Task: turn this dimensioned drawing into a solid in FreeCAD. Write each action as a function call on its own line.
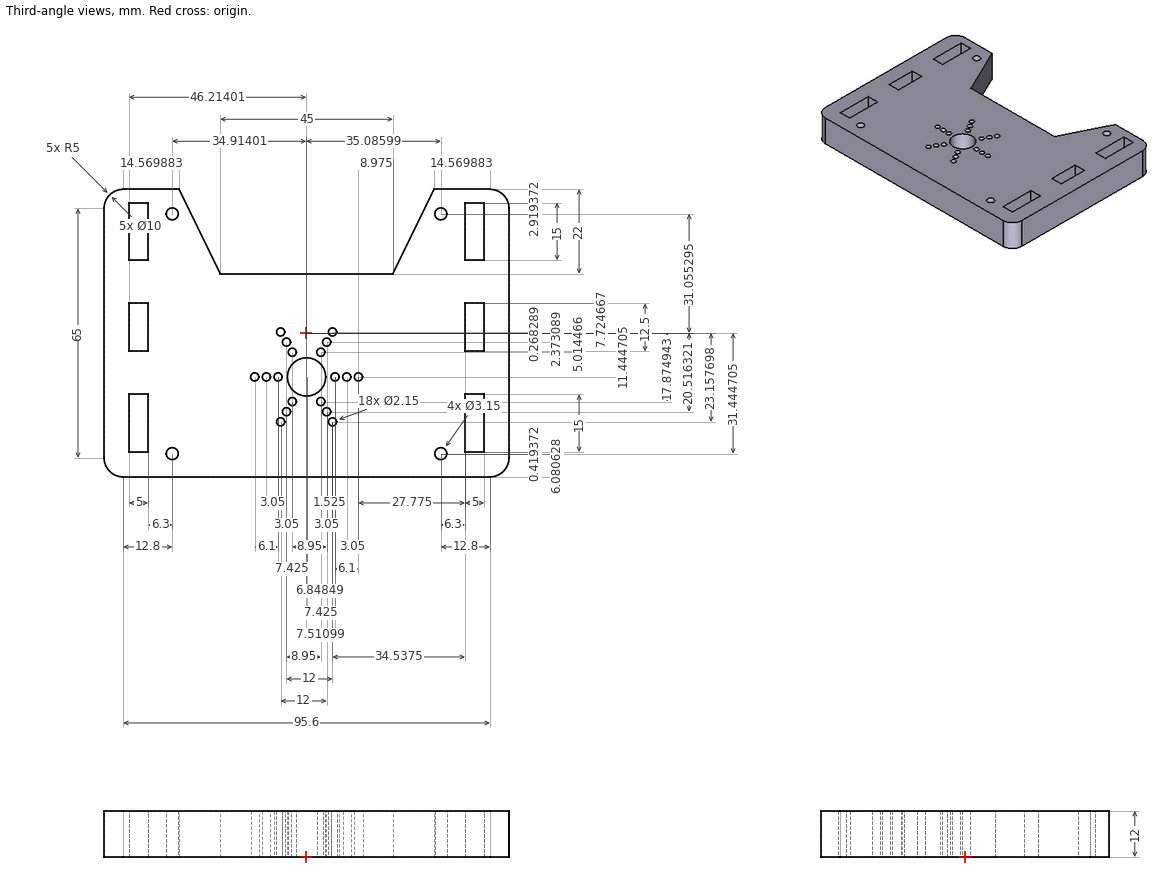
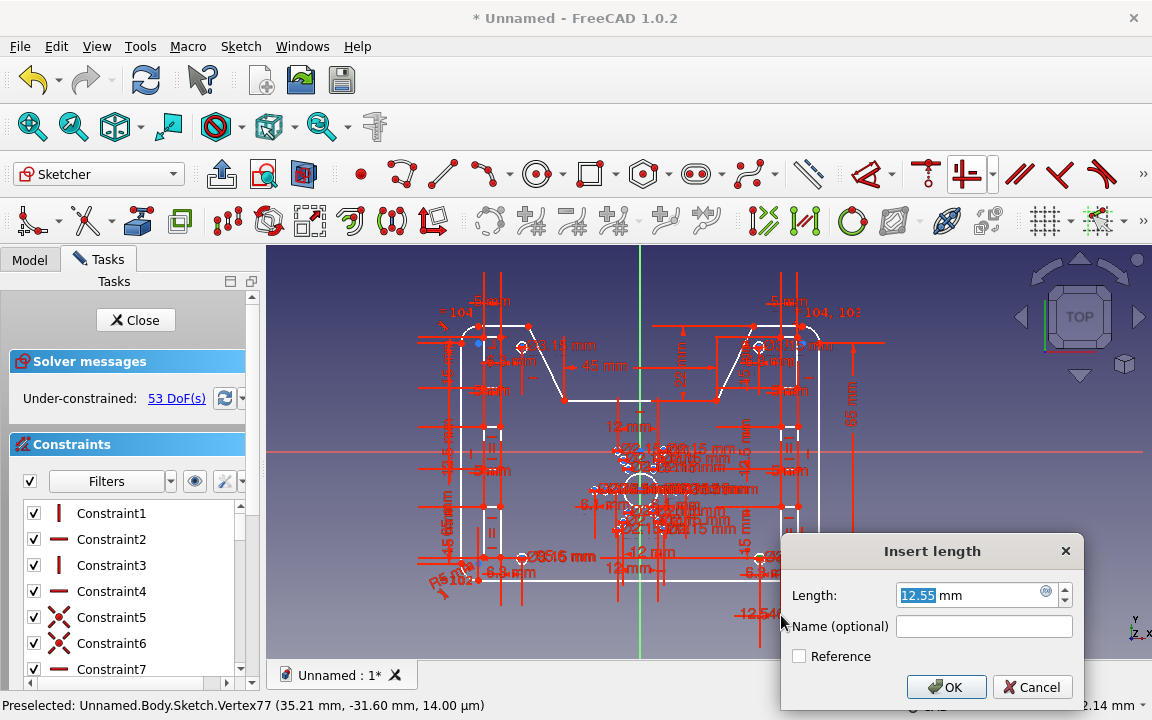
text(12.8)
key(Return)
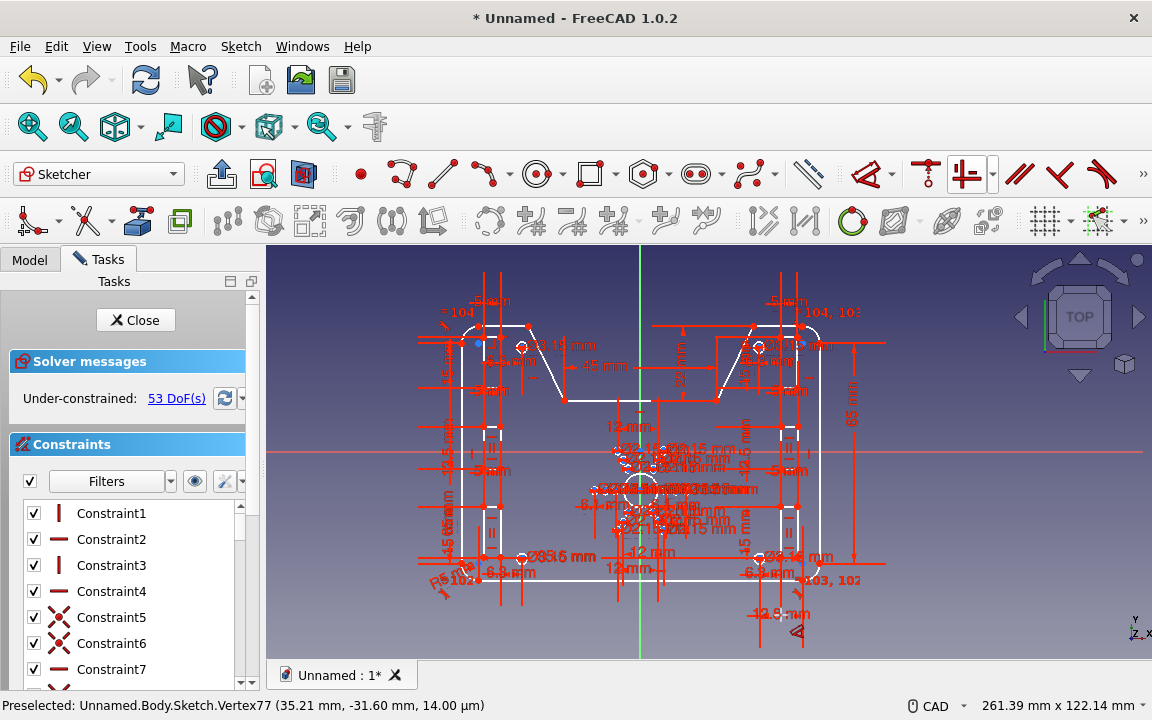
scroll(664, 531, up, 7)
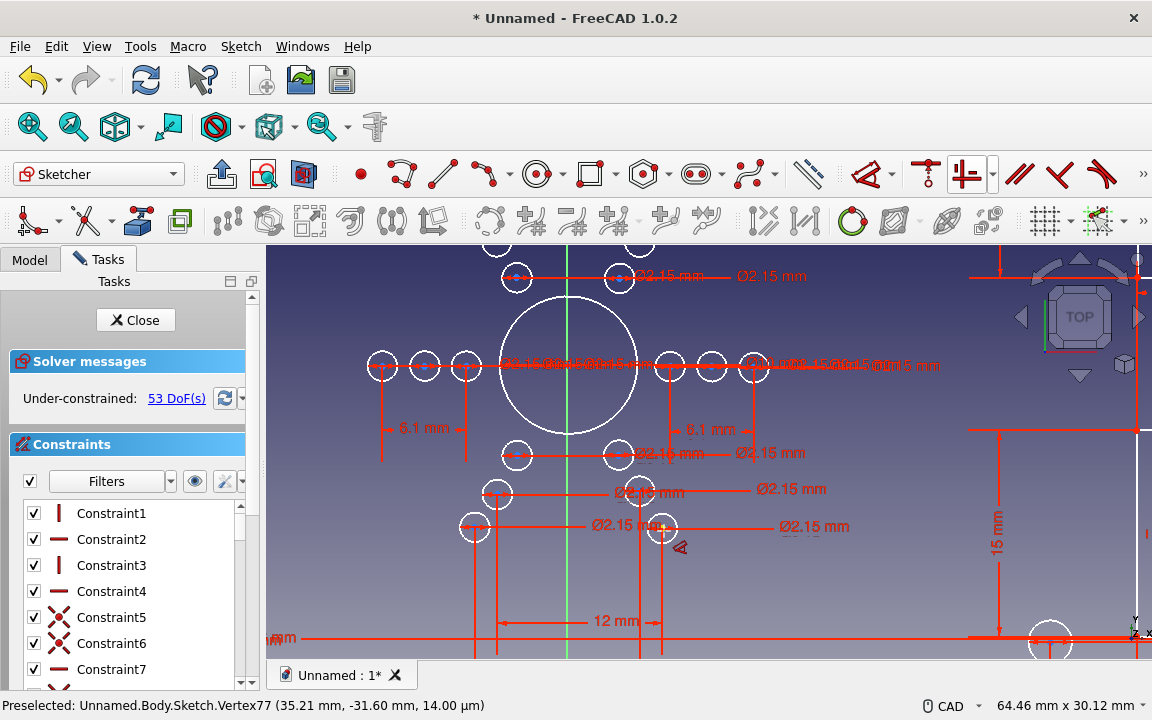
click(662, 529)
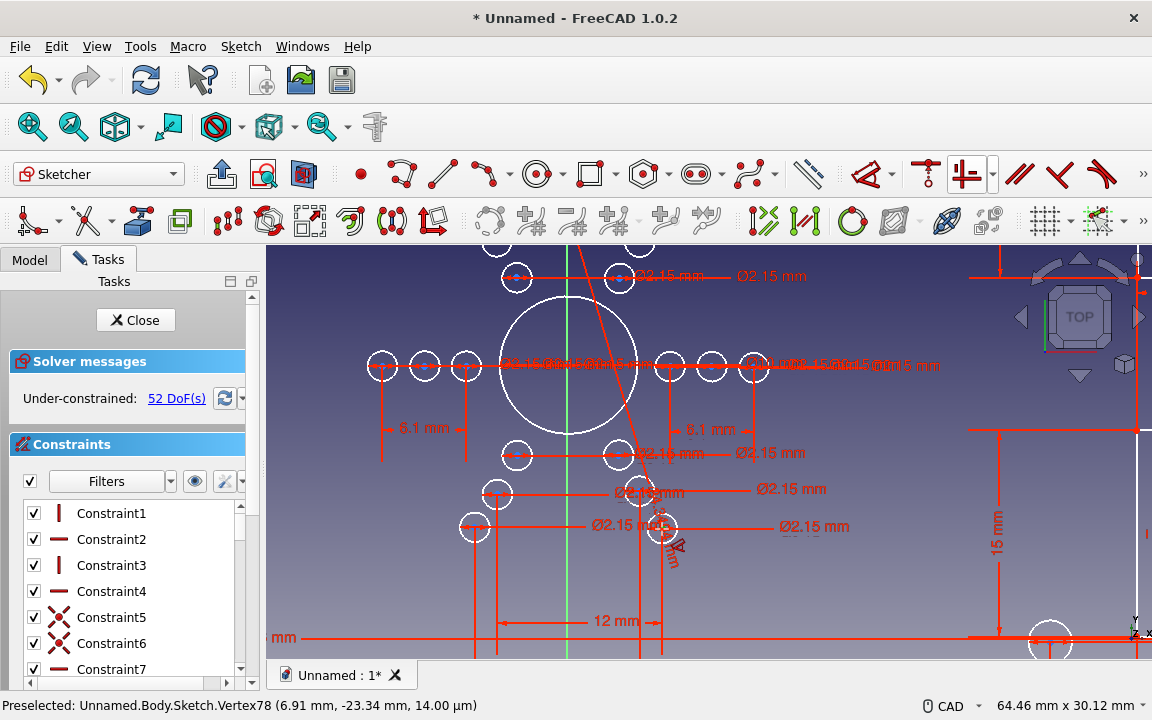
click(619, 455)
click(641, 563)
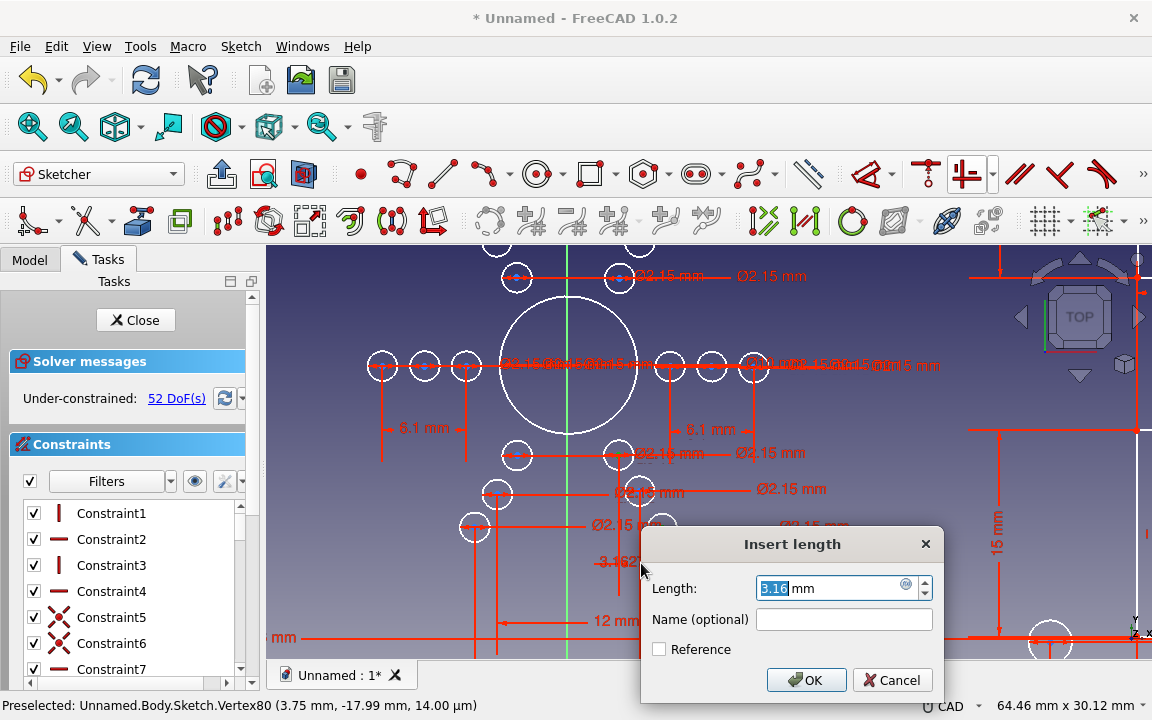
text(3.05)
key(Return)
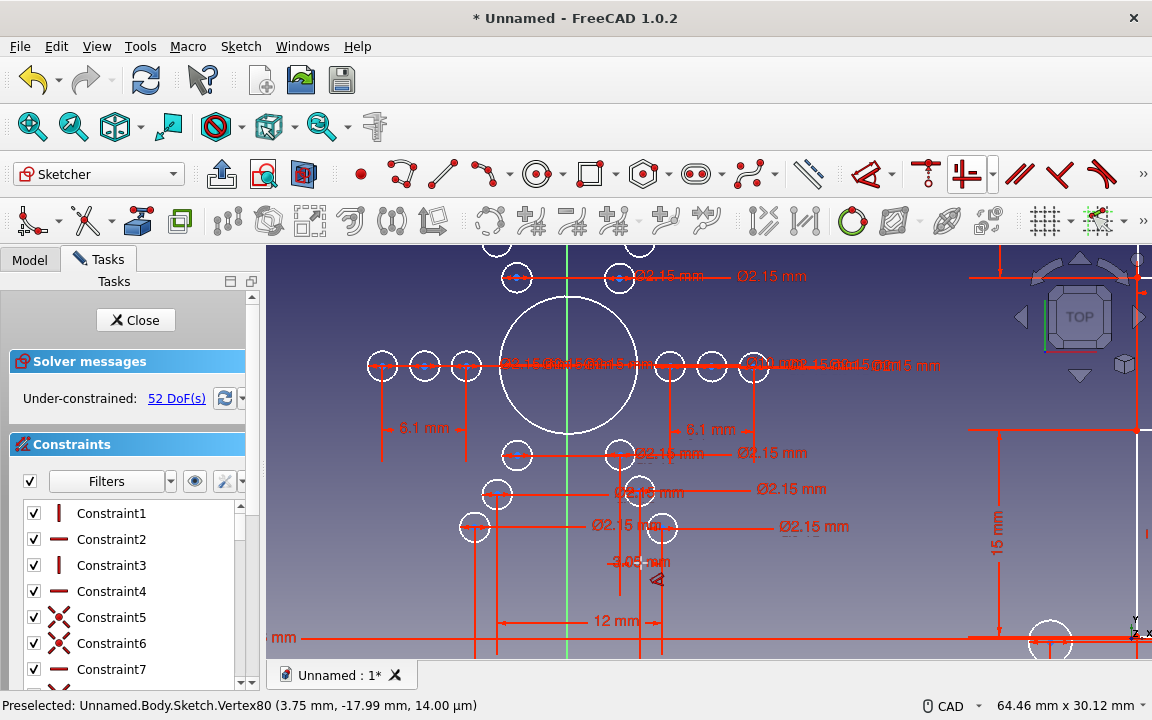
click(754, 368)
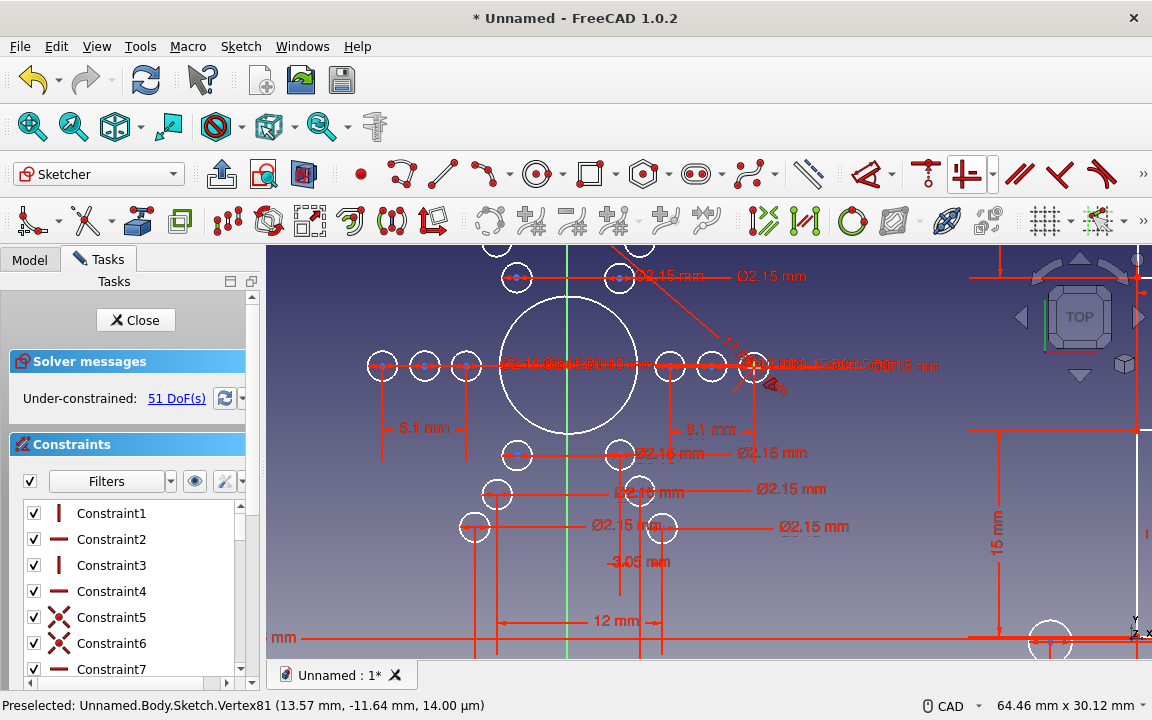
click(712, 367)
click(733, 402)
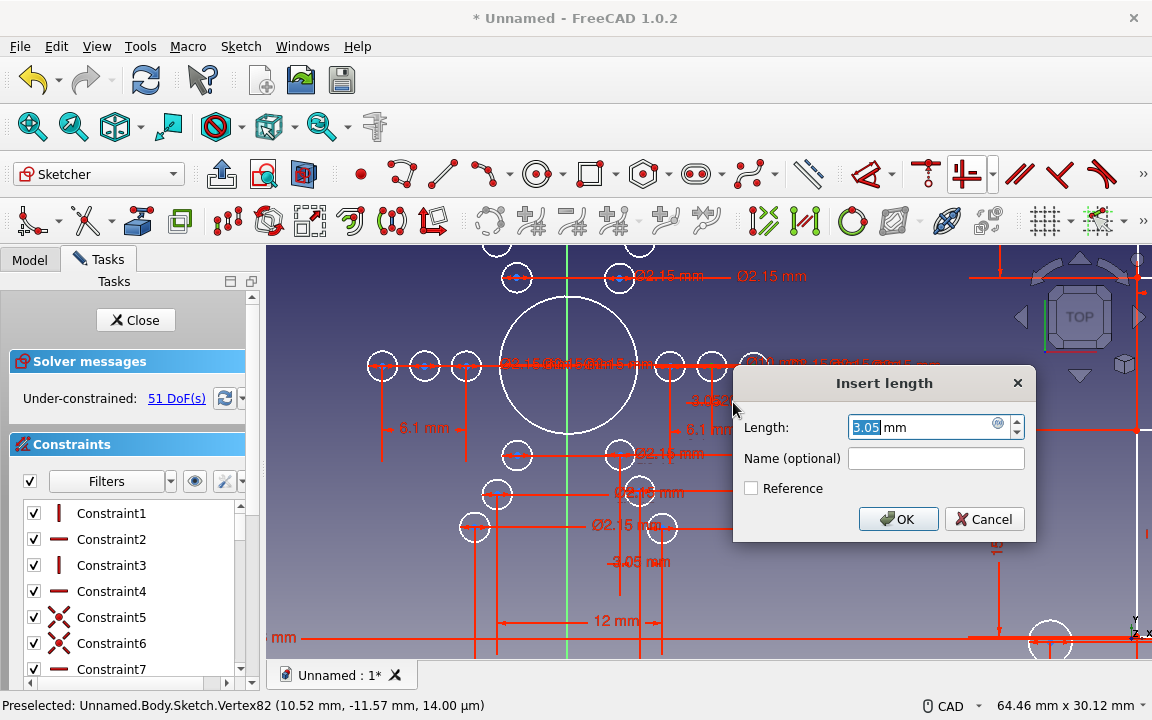
text(3.05)
key(Return)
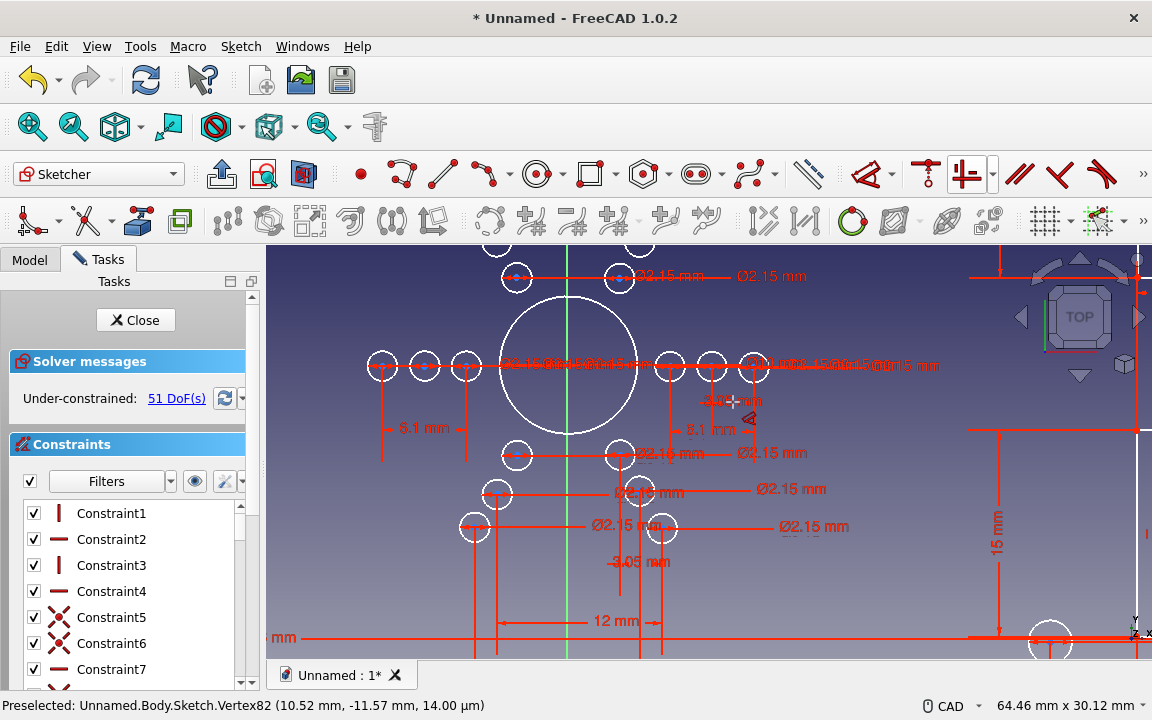
click(662, 529)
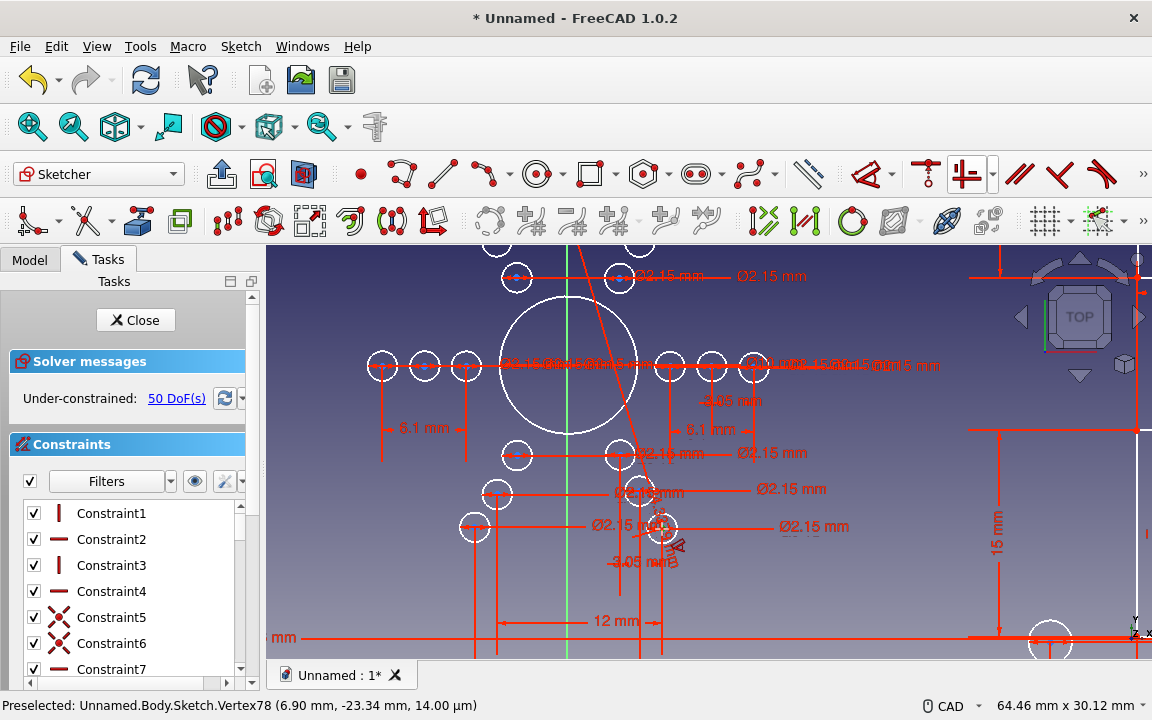
click(620, 278)
click(641, 587)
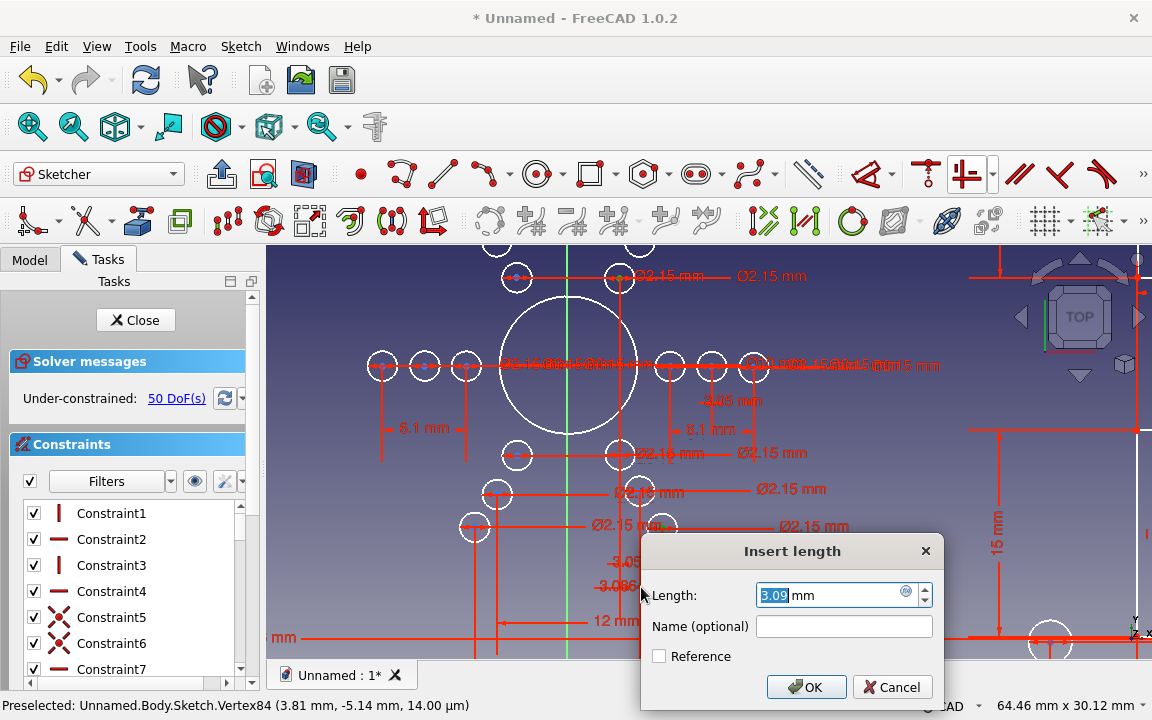
text(3.05)
key(Return)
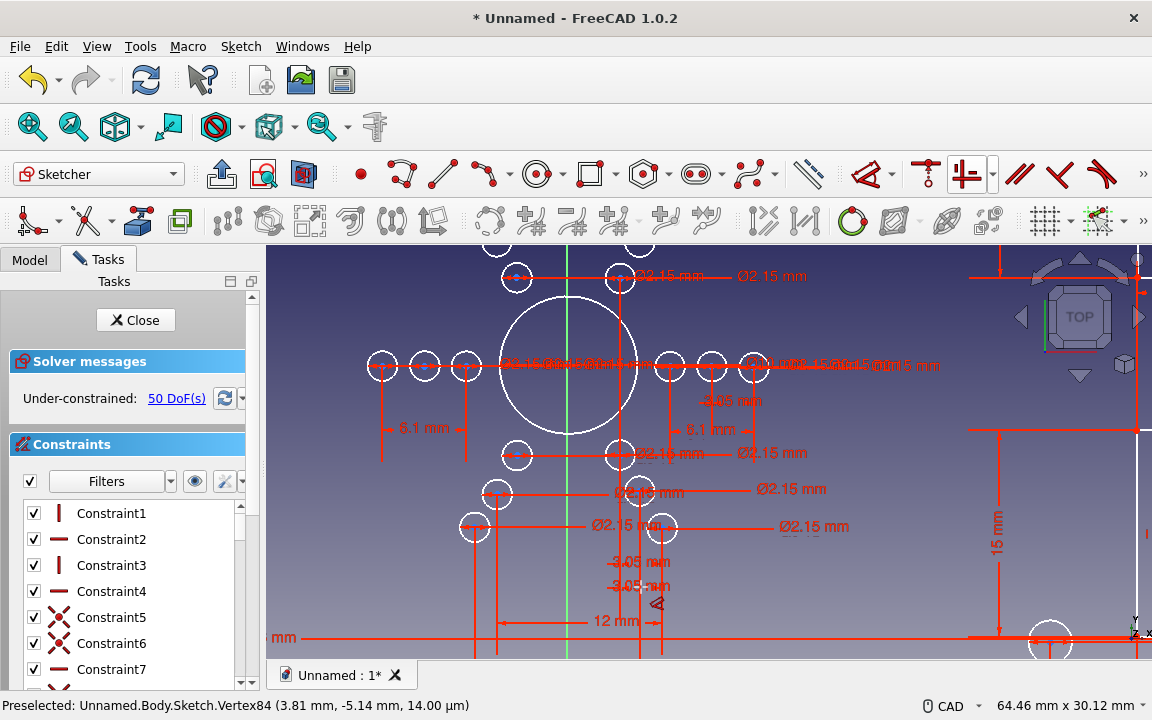
click(620, 278)